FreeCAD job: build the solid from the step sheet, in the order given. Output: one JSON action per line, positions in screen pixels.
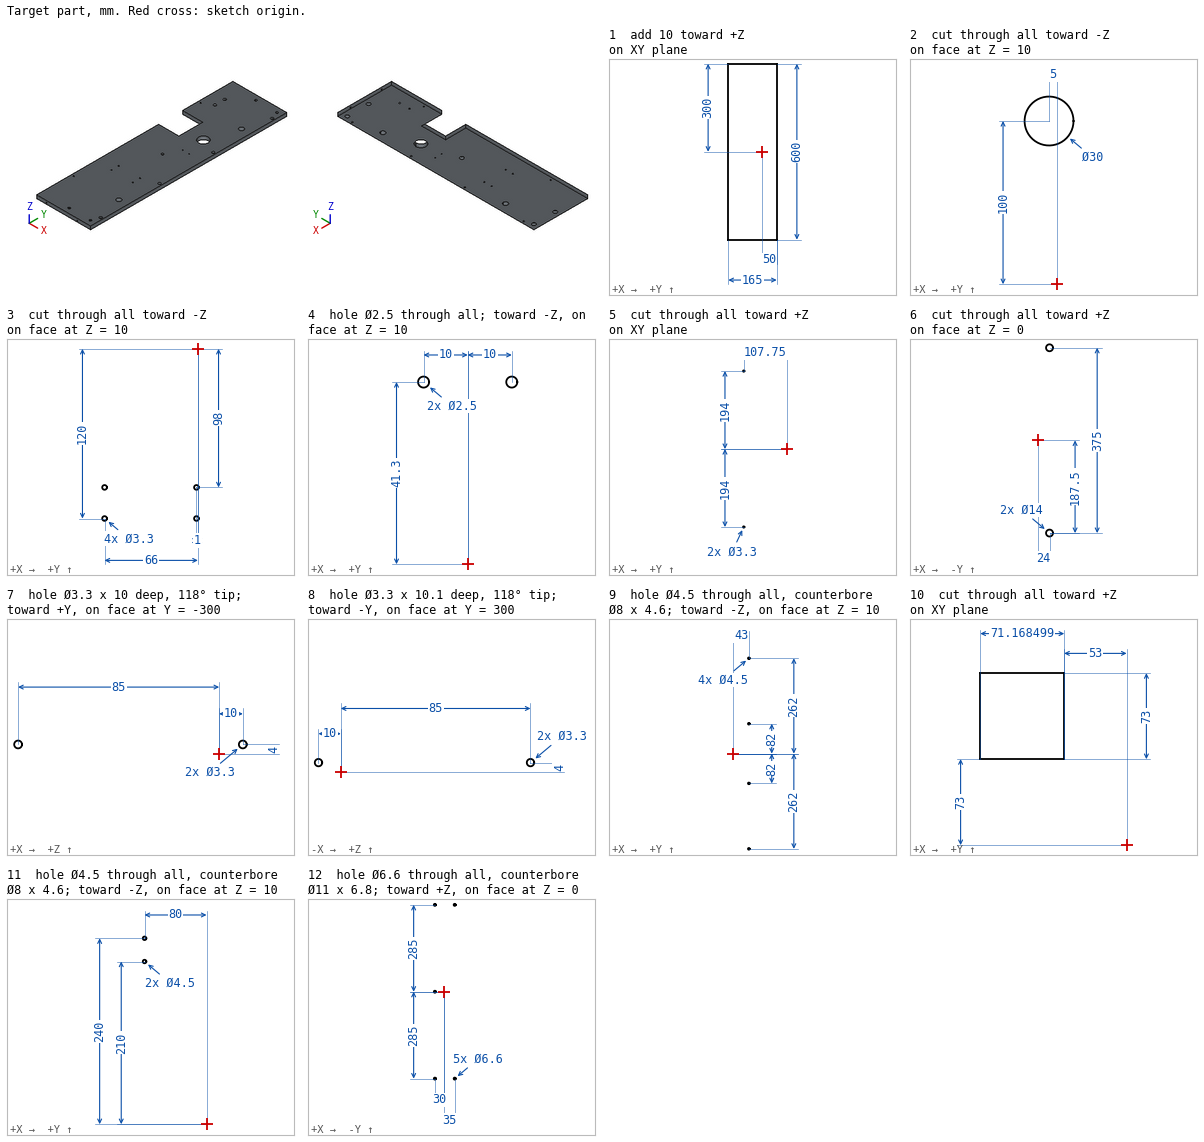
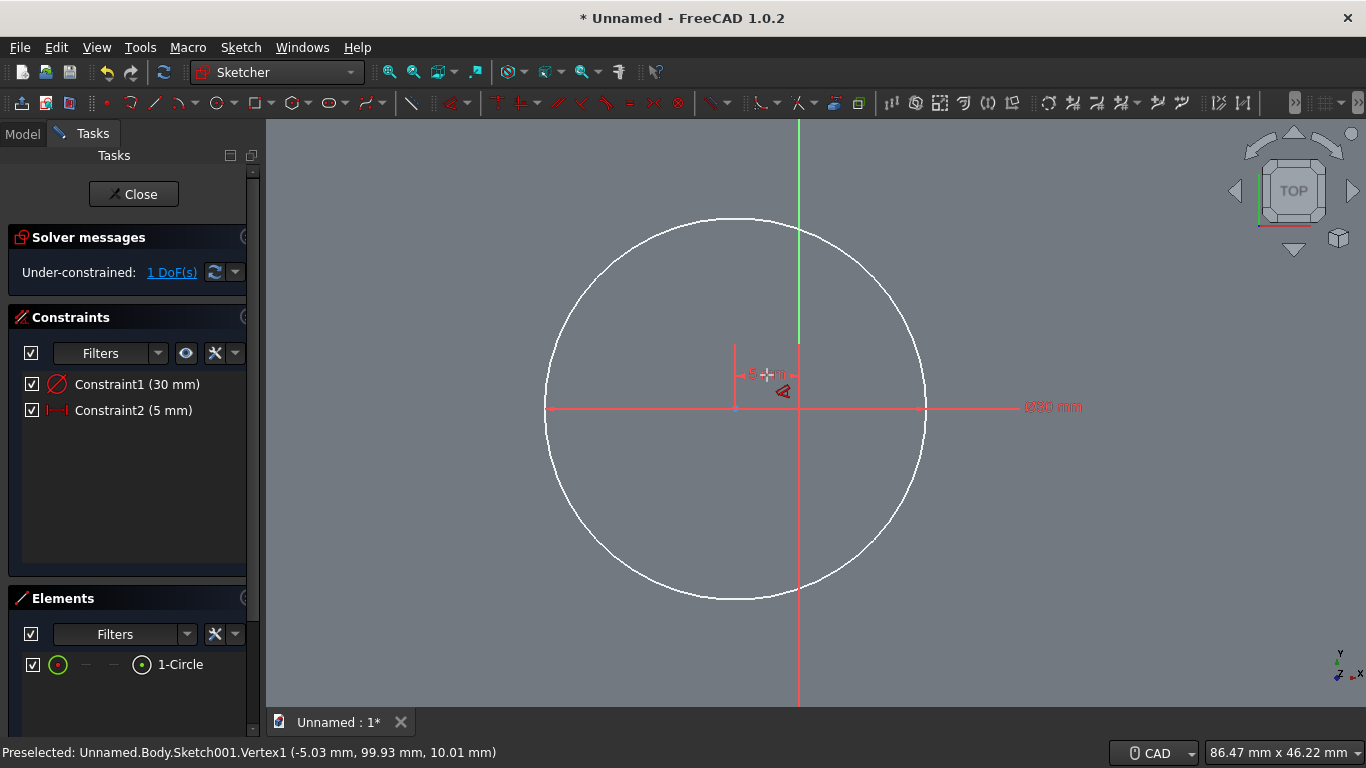
{"action": "left_click", "coordinate": [735, 409]}
{"action": "left_click", "coordinate": [833, 544]}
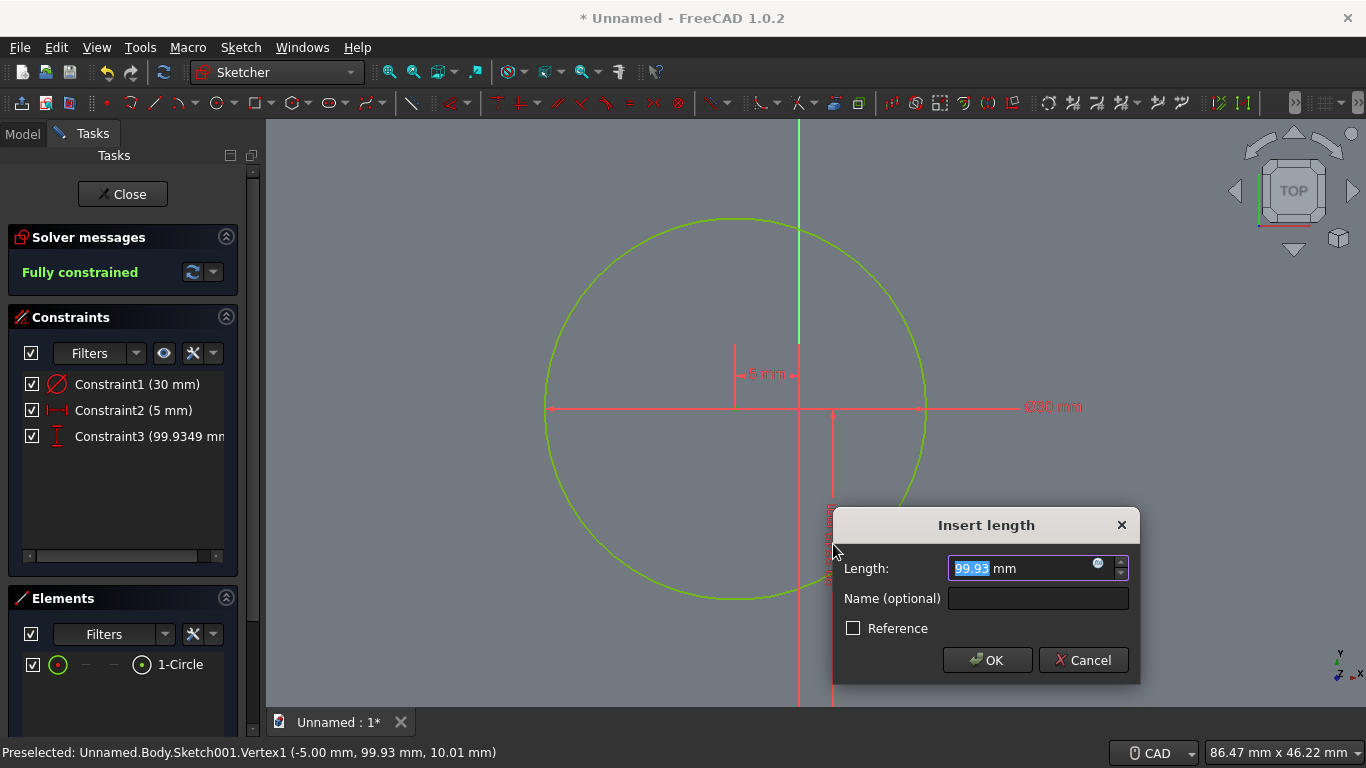
{"action": "type", "text": "100"}
{"action": "key", "text": "Return"}
{"action": "key", "text": "Escape"}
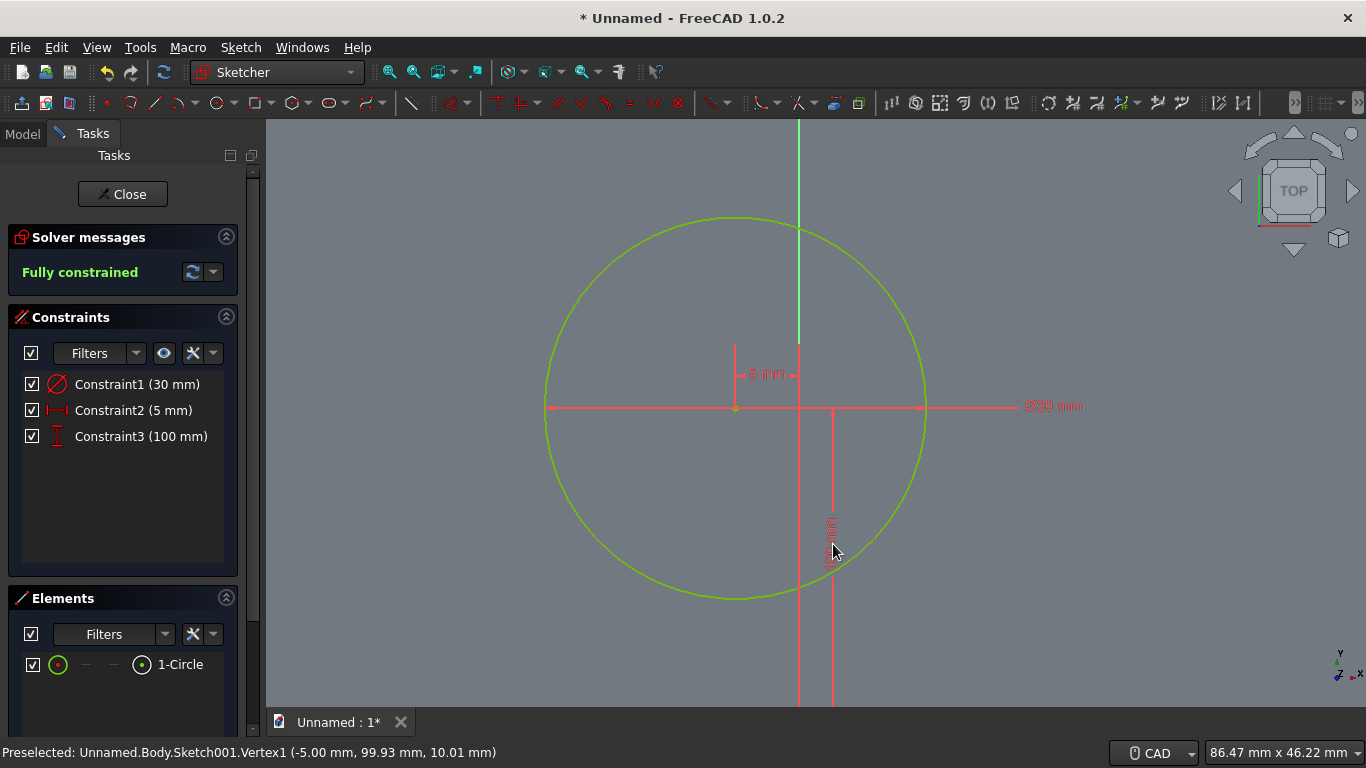
{"action": "left_click", "coordinate": [123, 194]}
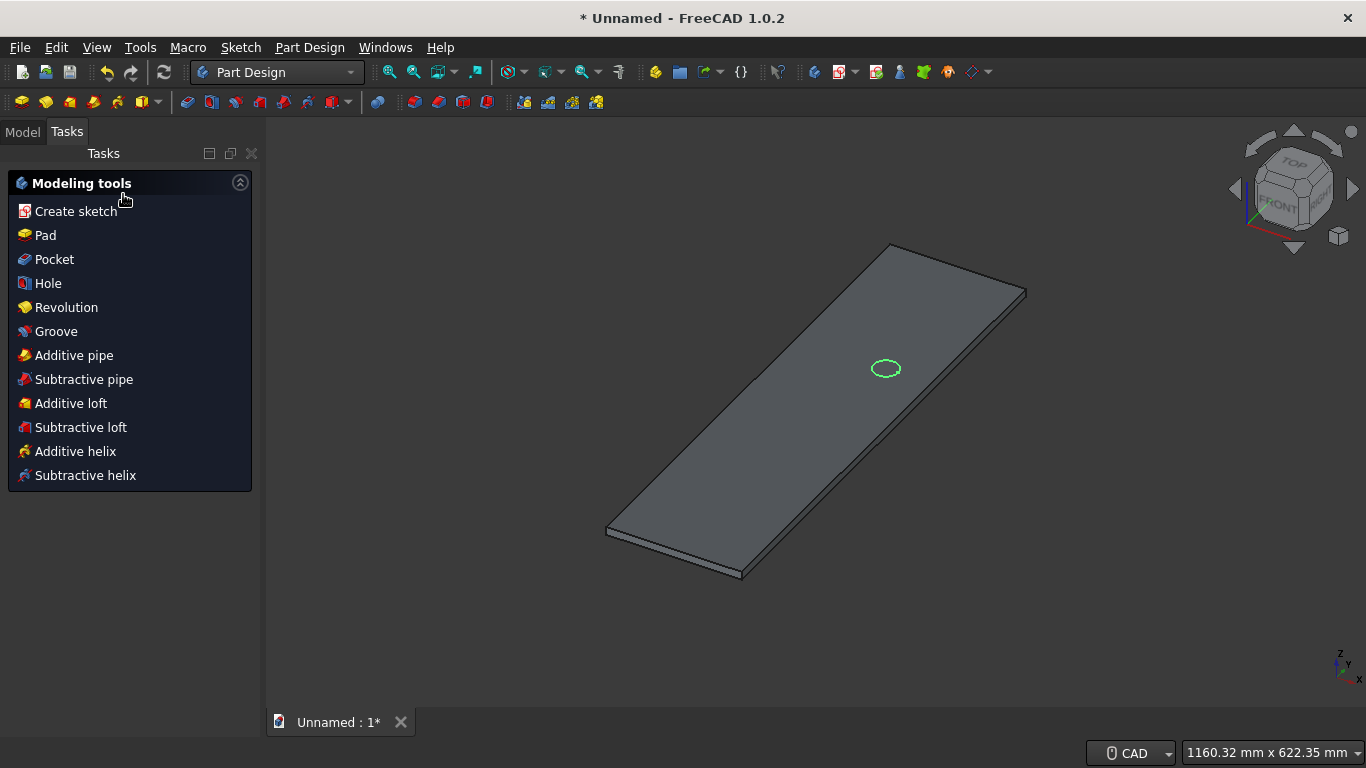
{"action": "left_click", "coordinate": [188, 102]}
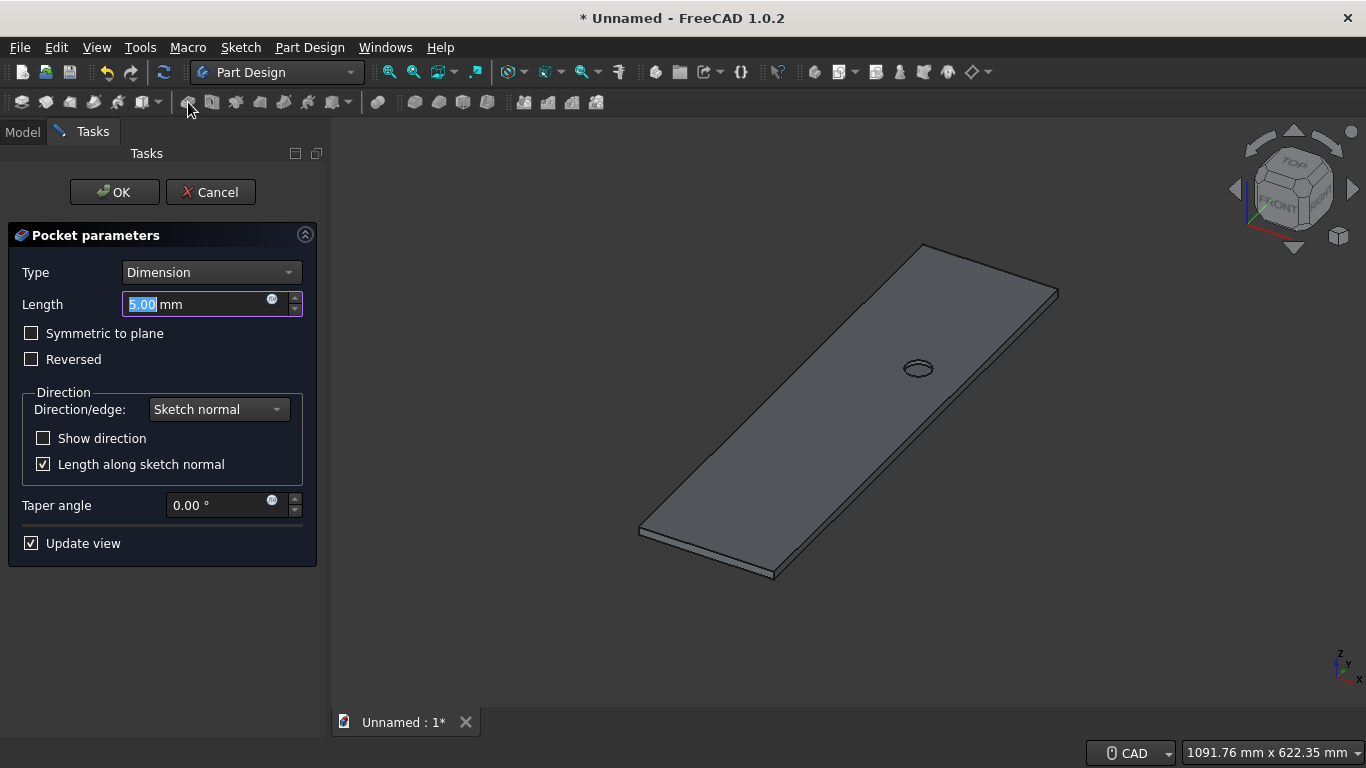
{"action": "left_click", "coordinate": [212, 272]}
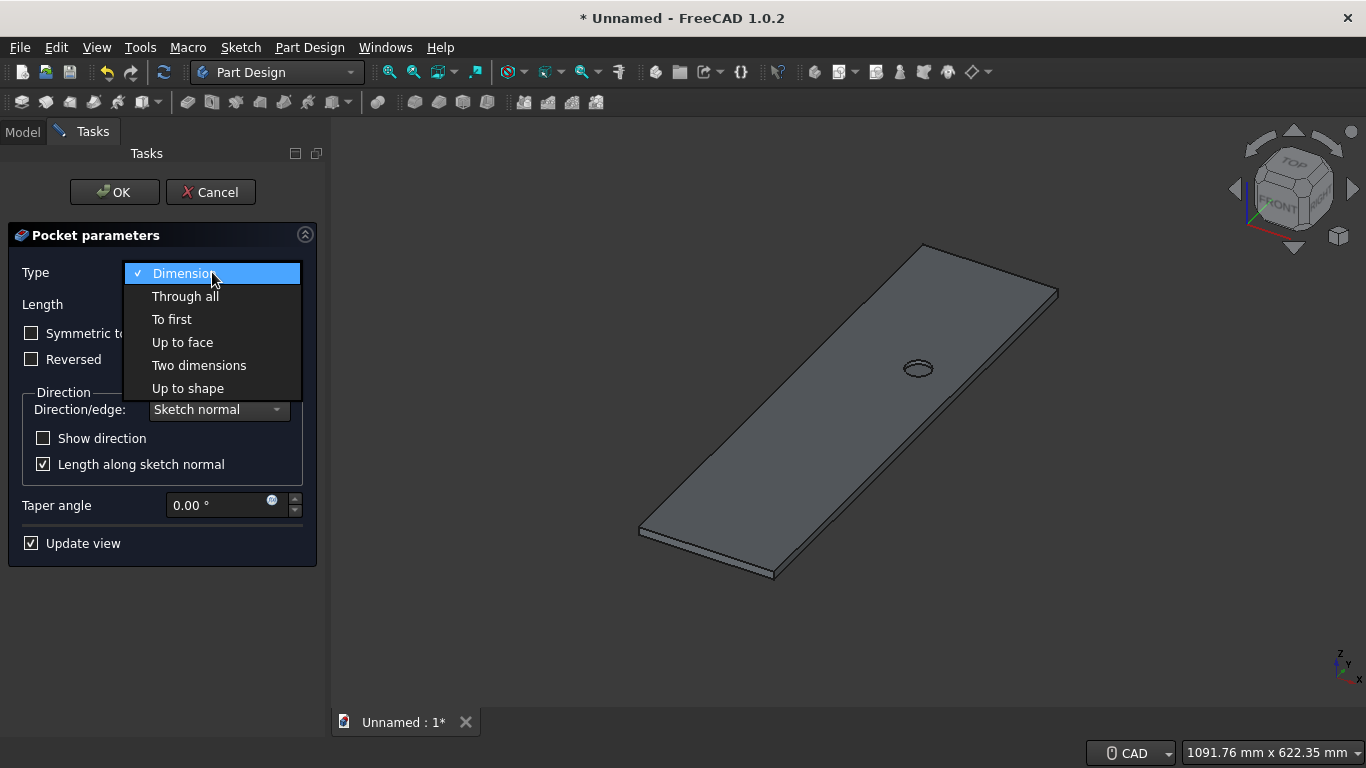
{"action": "left_click", "coordinate": [212, 296]}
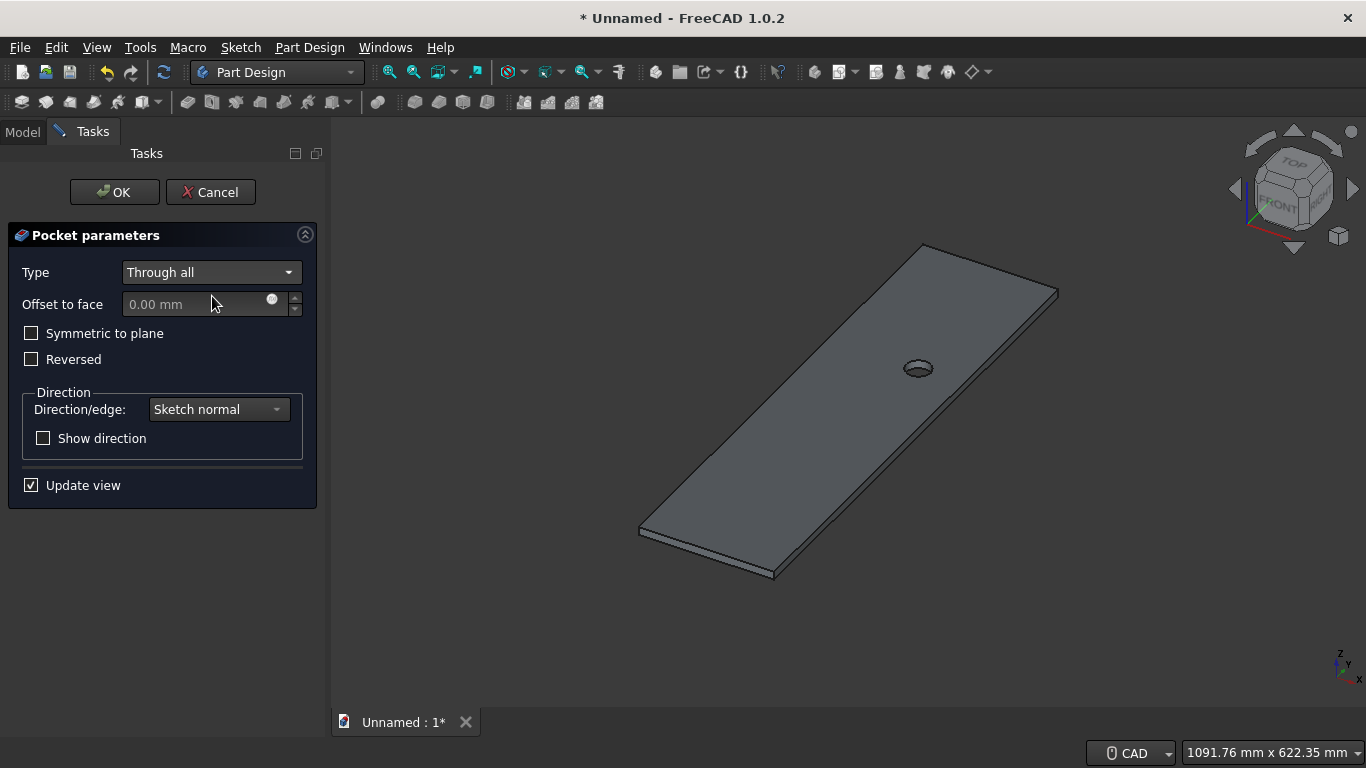
{"action": "left_click", "coordinate": [115, 192]}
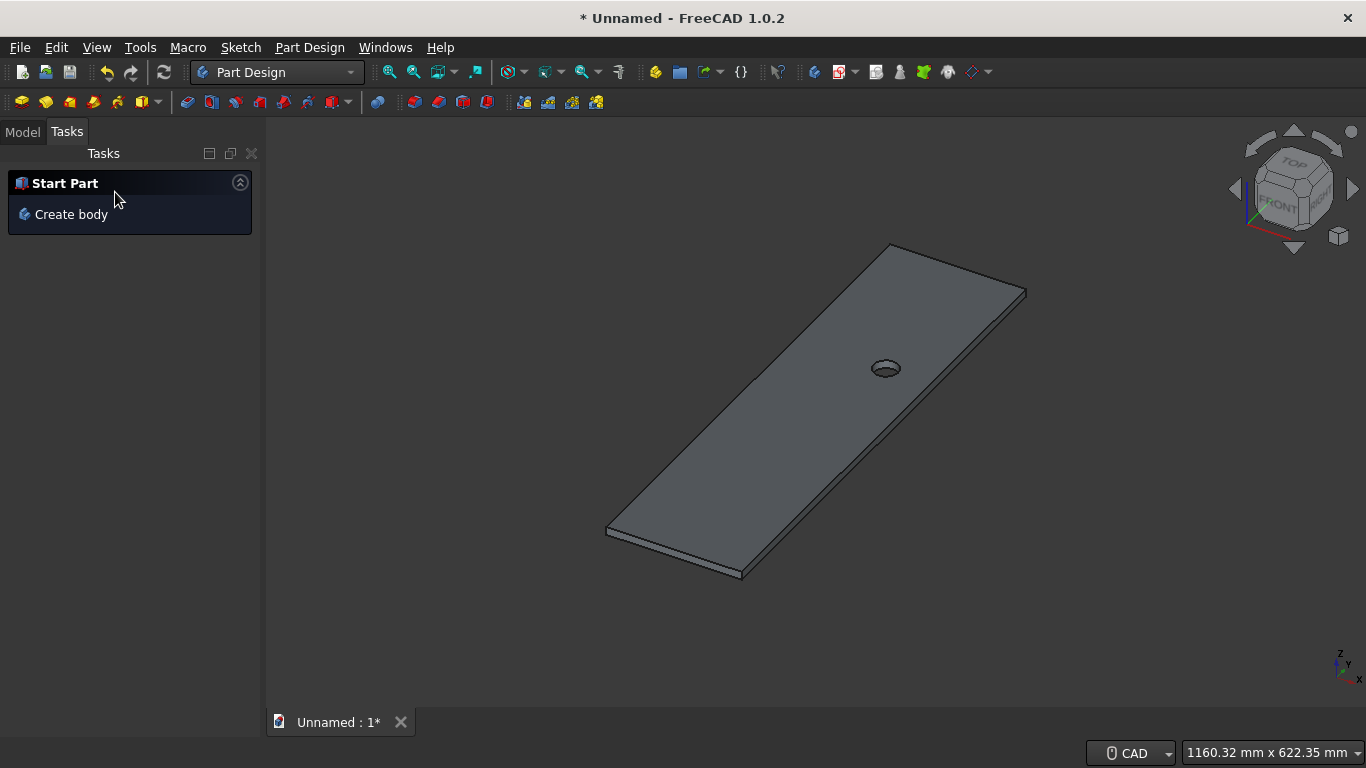
{"action": "left_click", "coordinate": [816, 407]}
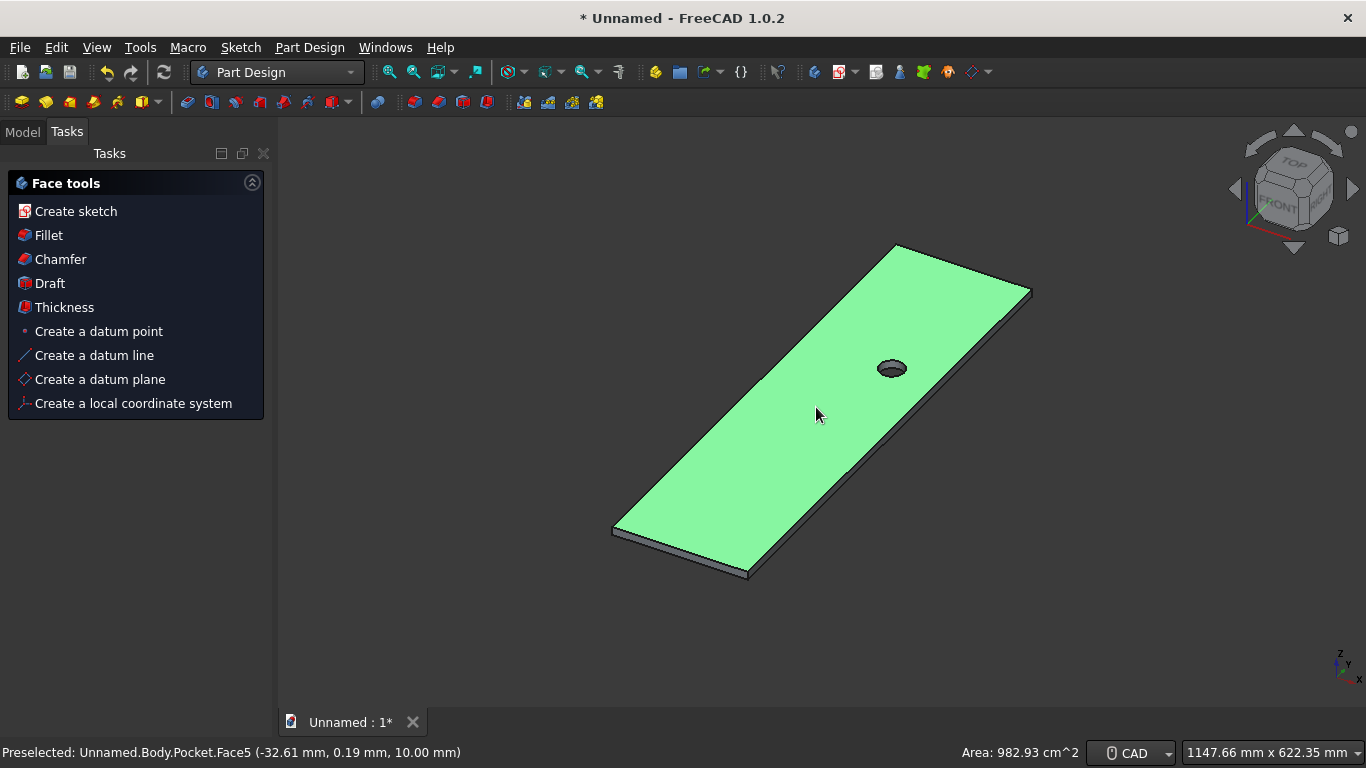
{"action": "left_click", "coordinate": [840, 72]}